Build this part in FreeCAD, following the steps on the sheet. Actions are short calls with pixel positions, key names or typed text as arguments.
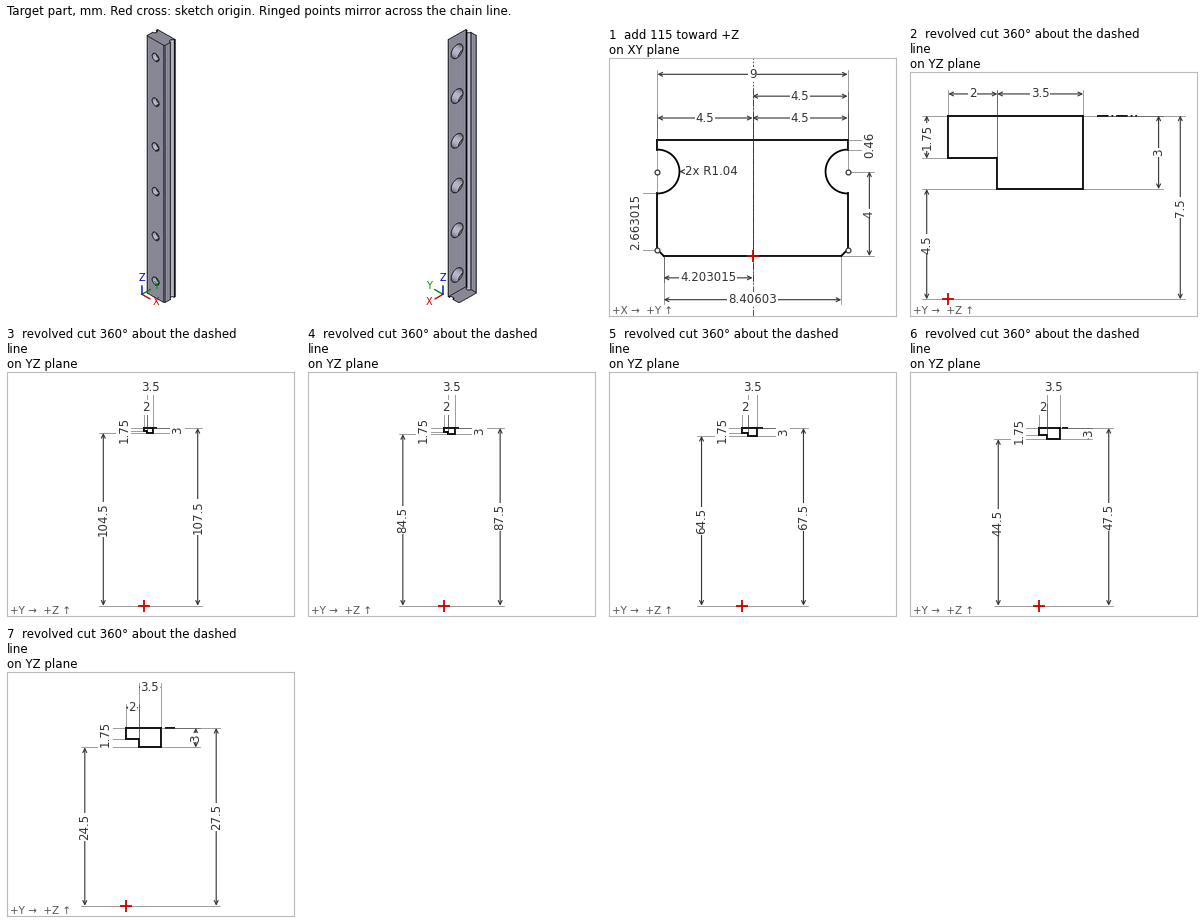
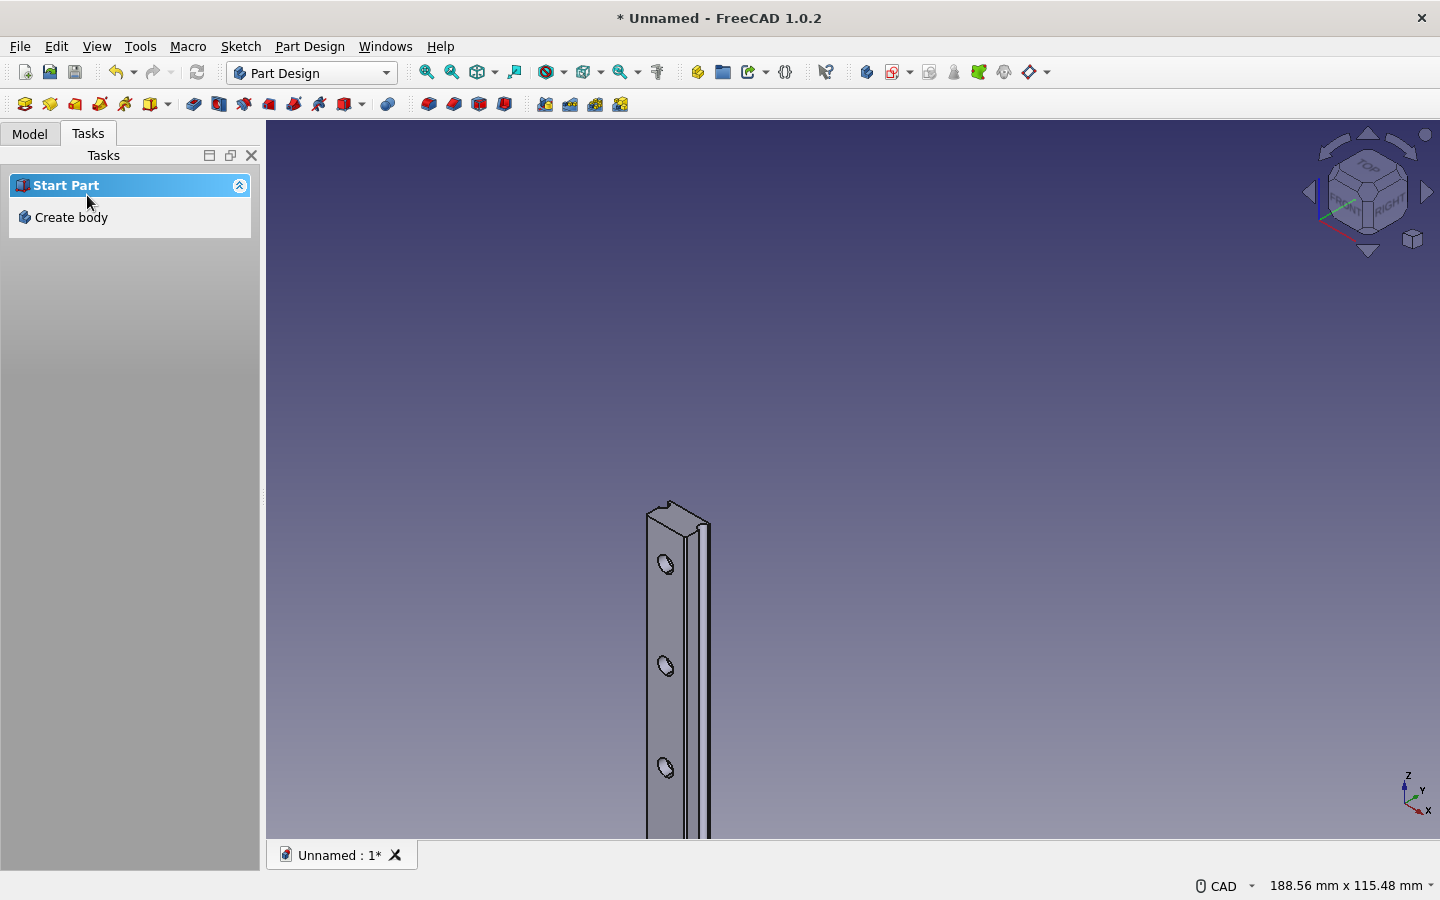
key(v)
key(f)